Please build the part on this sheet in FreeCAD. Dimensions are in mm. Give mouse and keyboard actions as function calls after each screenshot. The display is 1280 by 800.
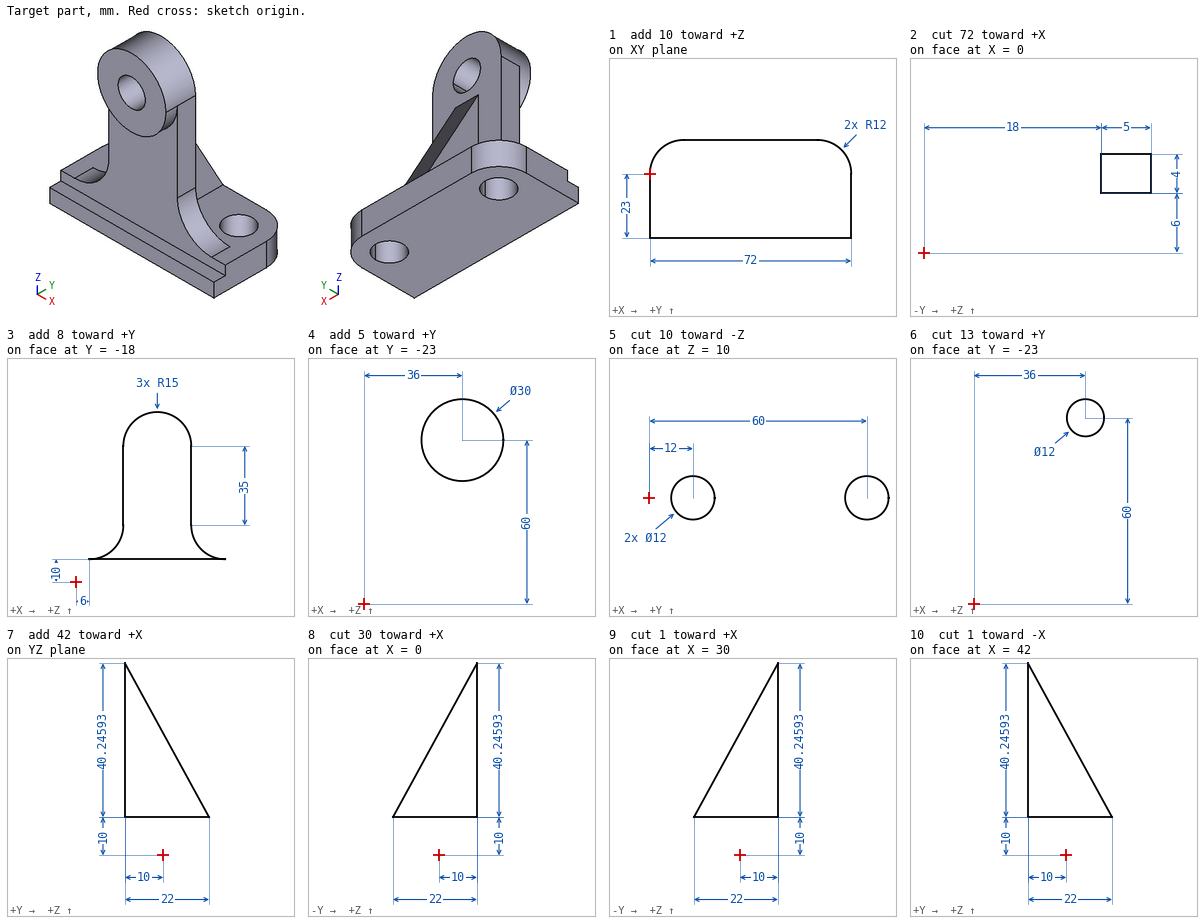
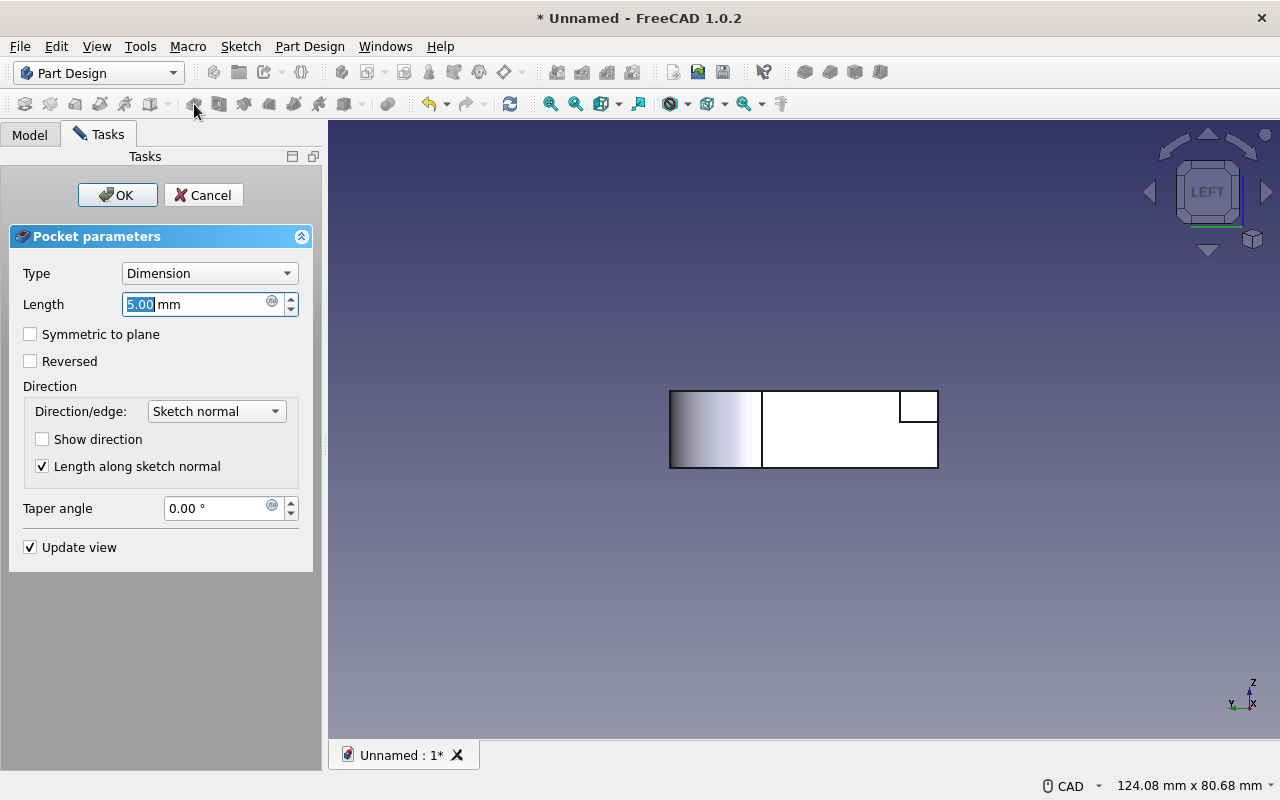
text(72)
key(Tab)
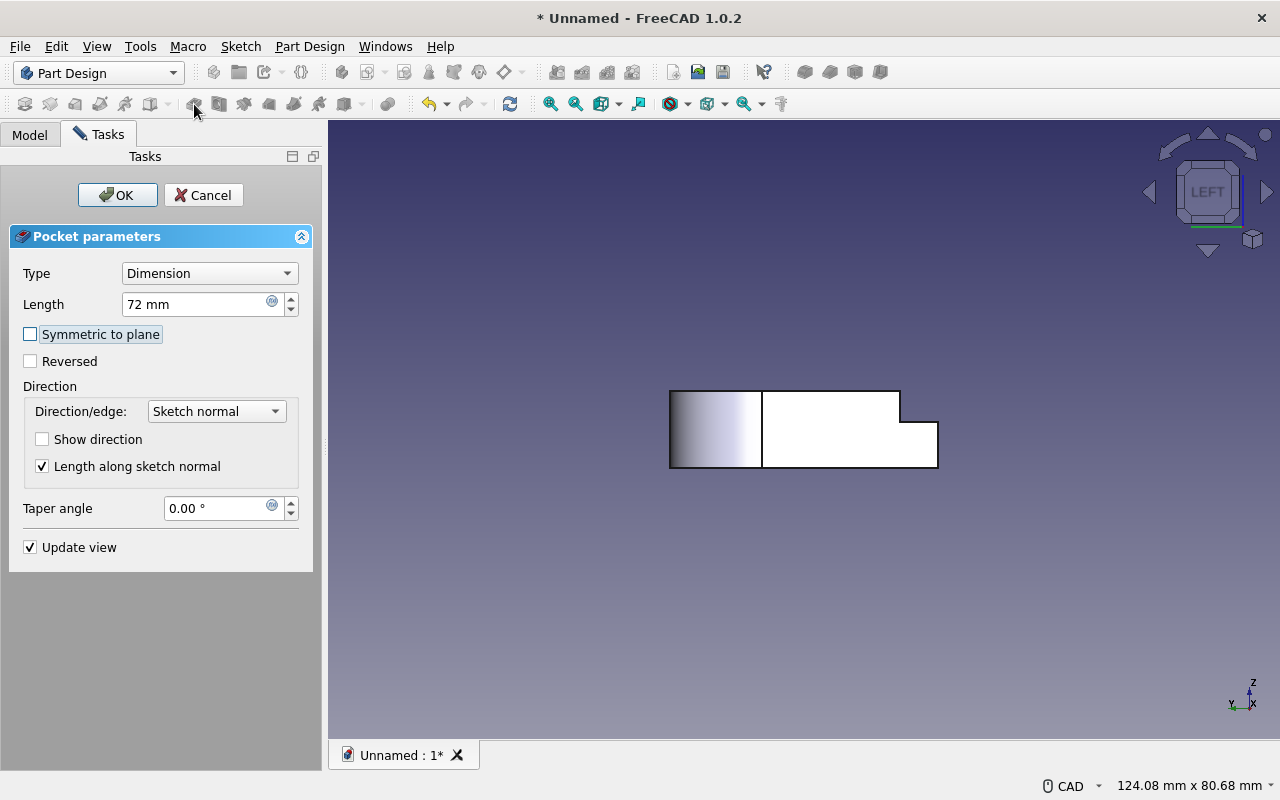
click(118, 195)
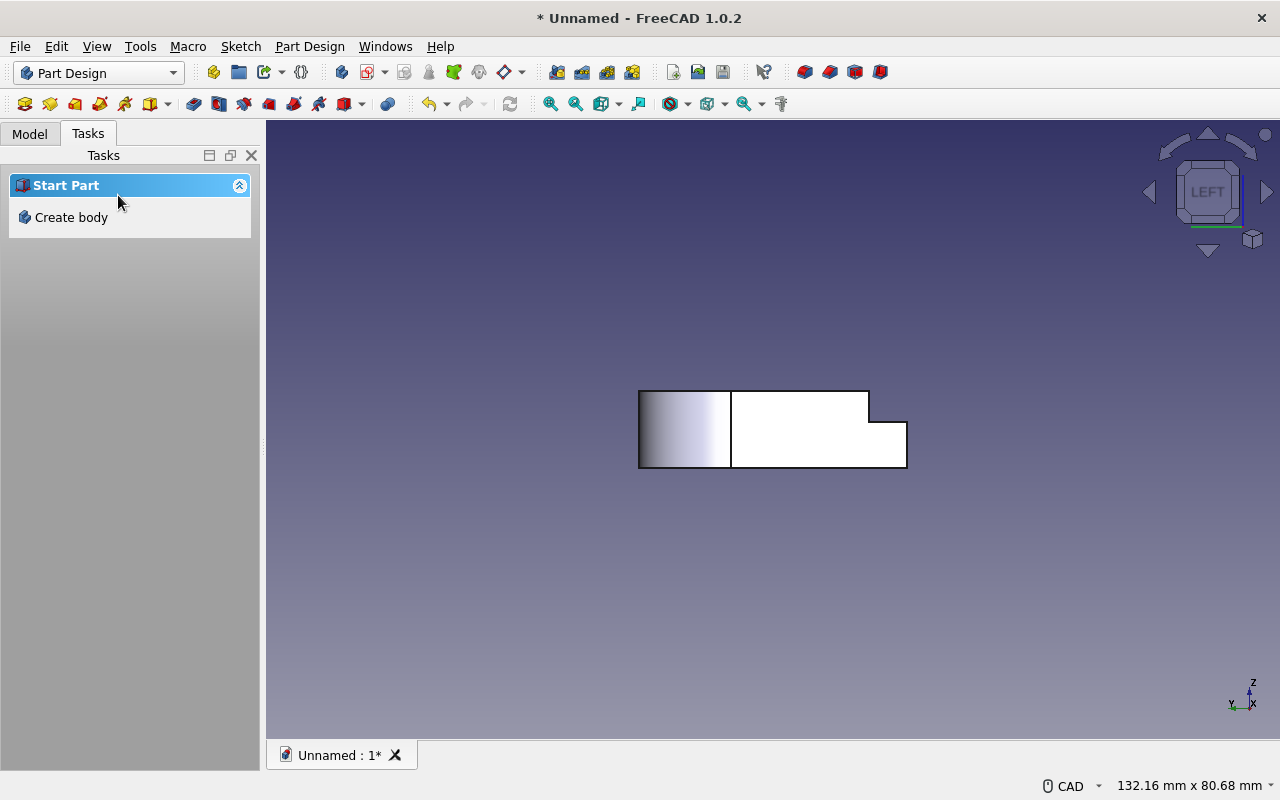
click(551, 104)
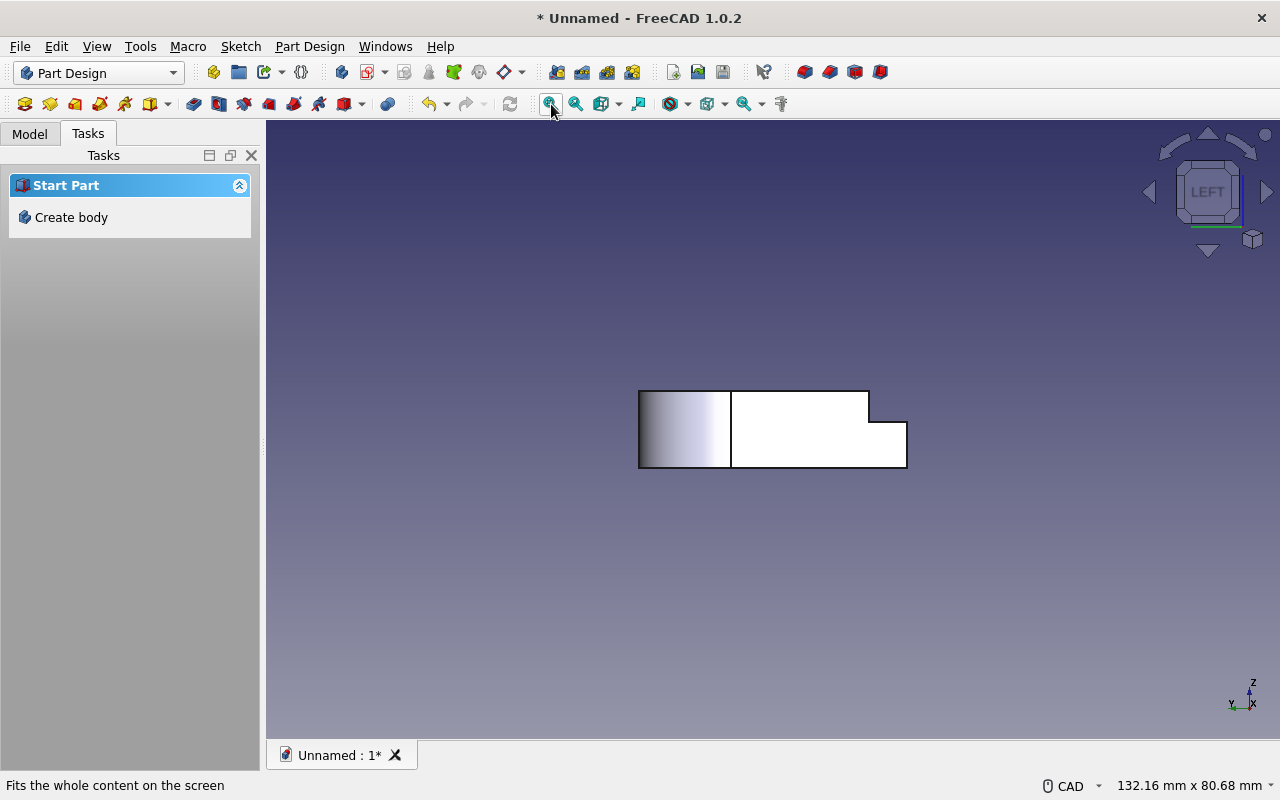
key(0)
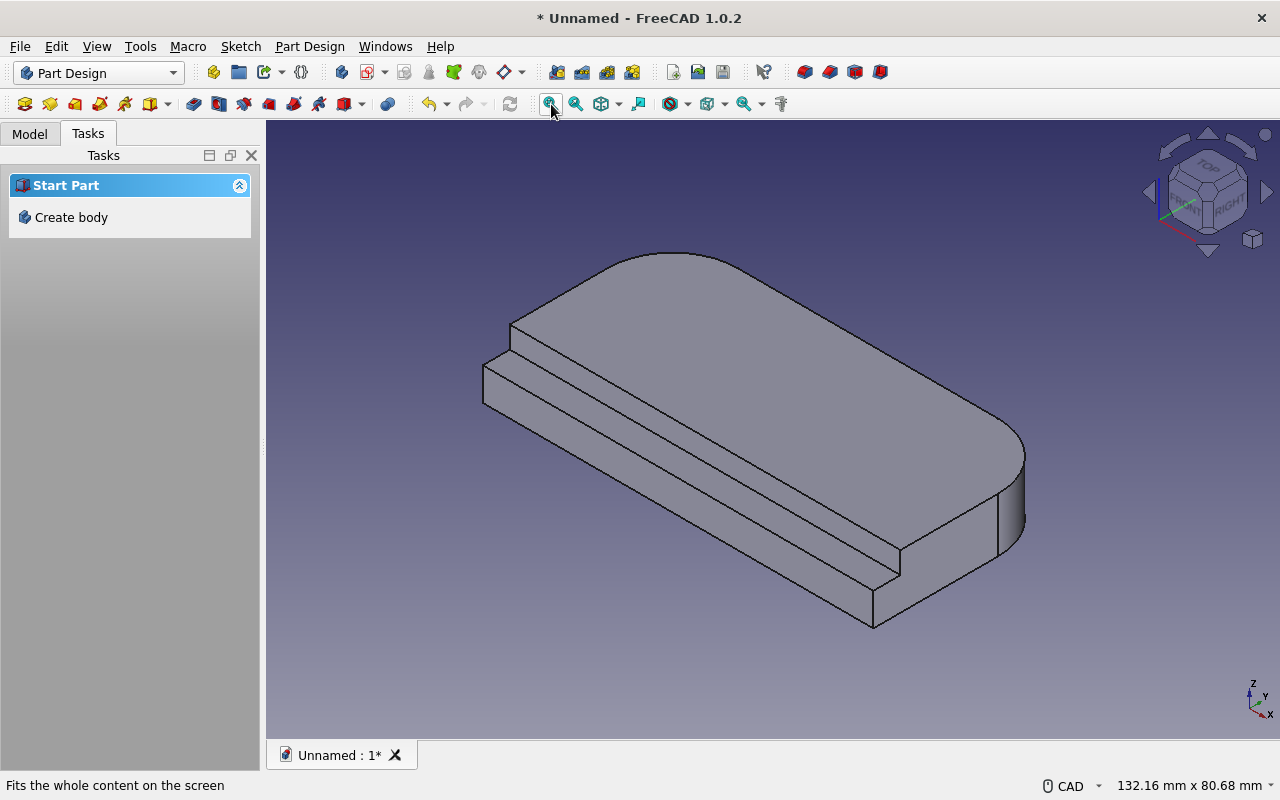
click(873, 546)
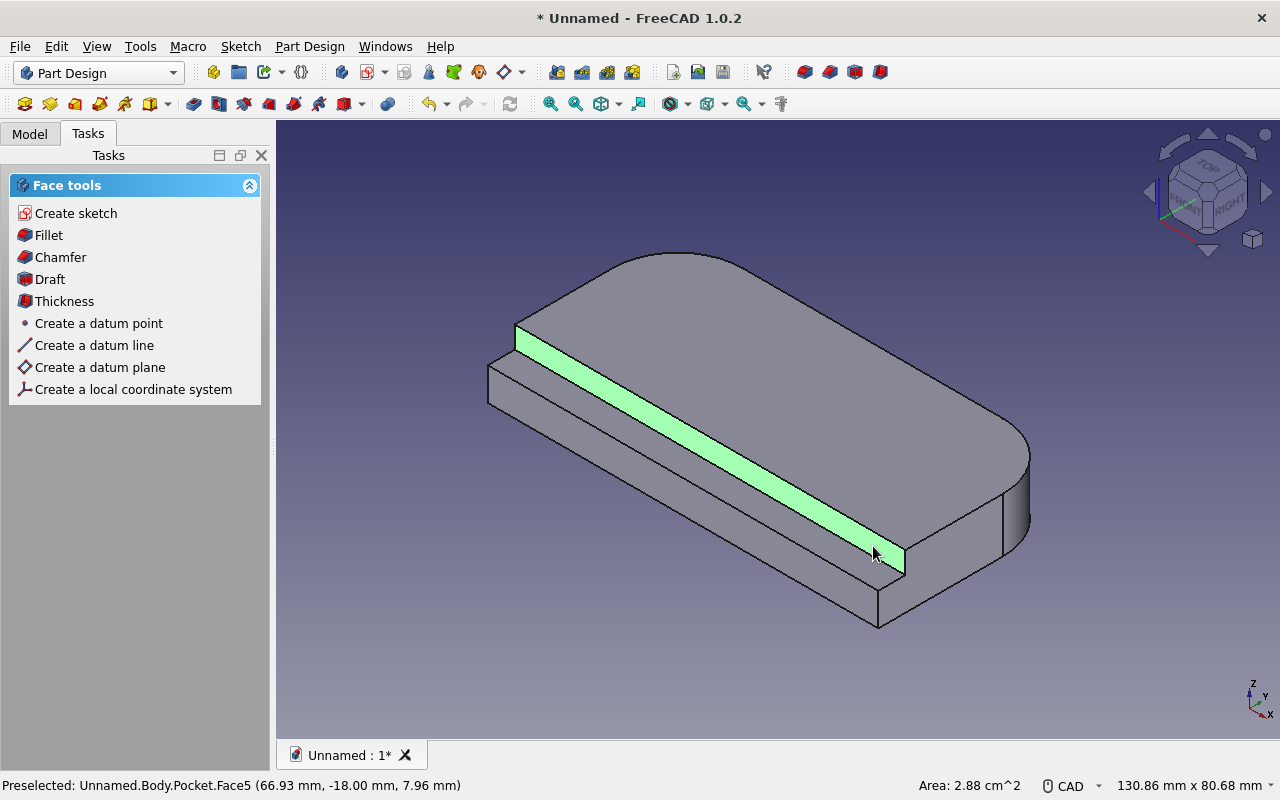
click(366, 72)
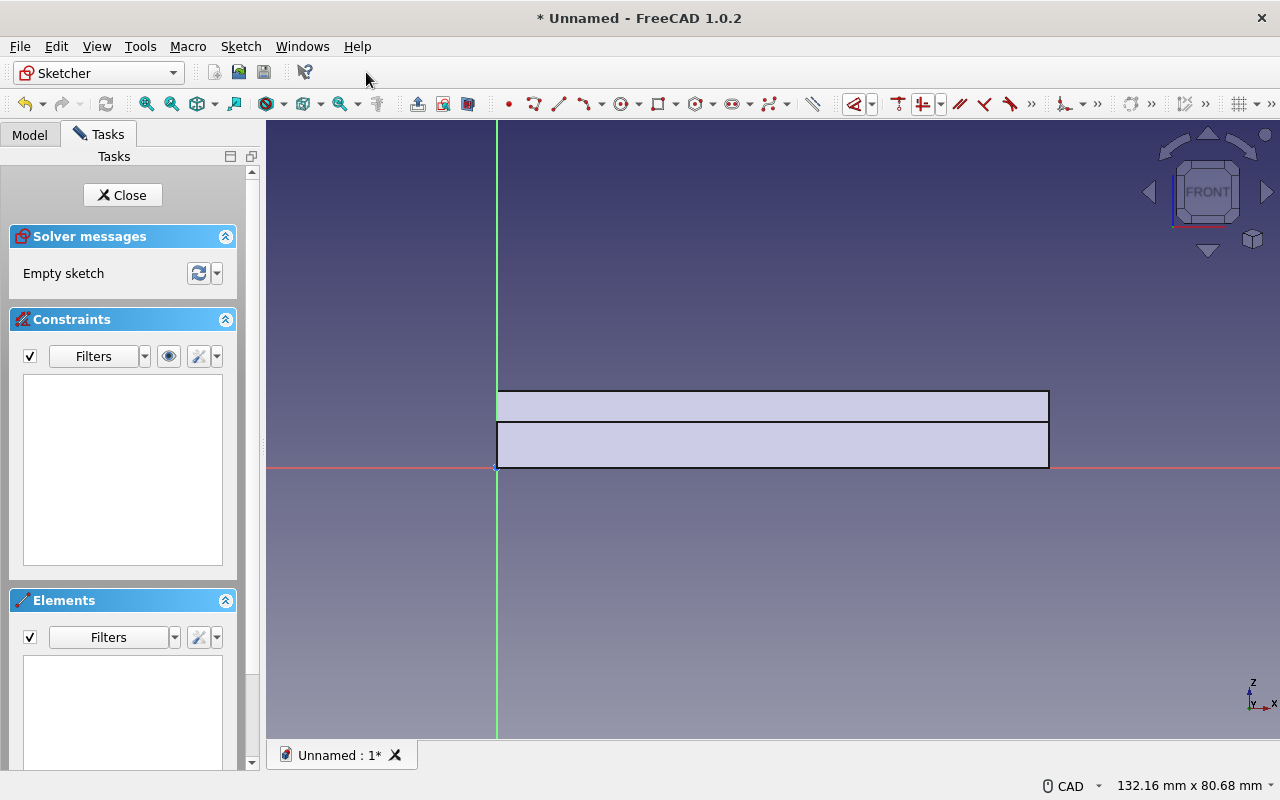
key(q)
key(s)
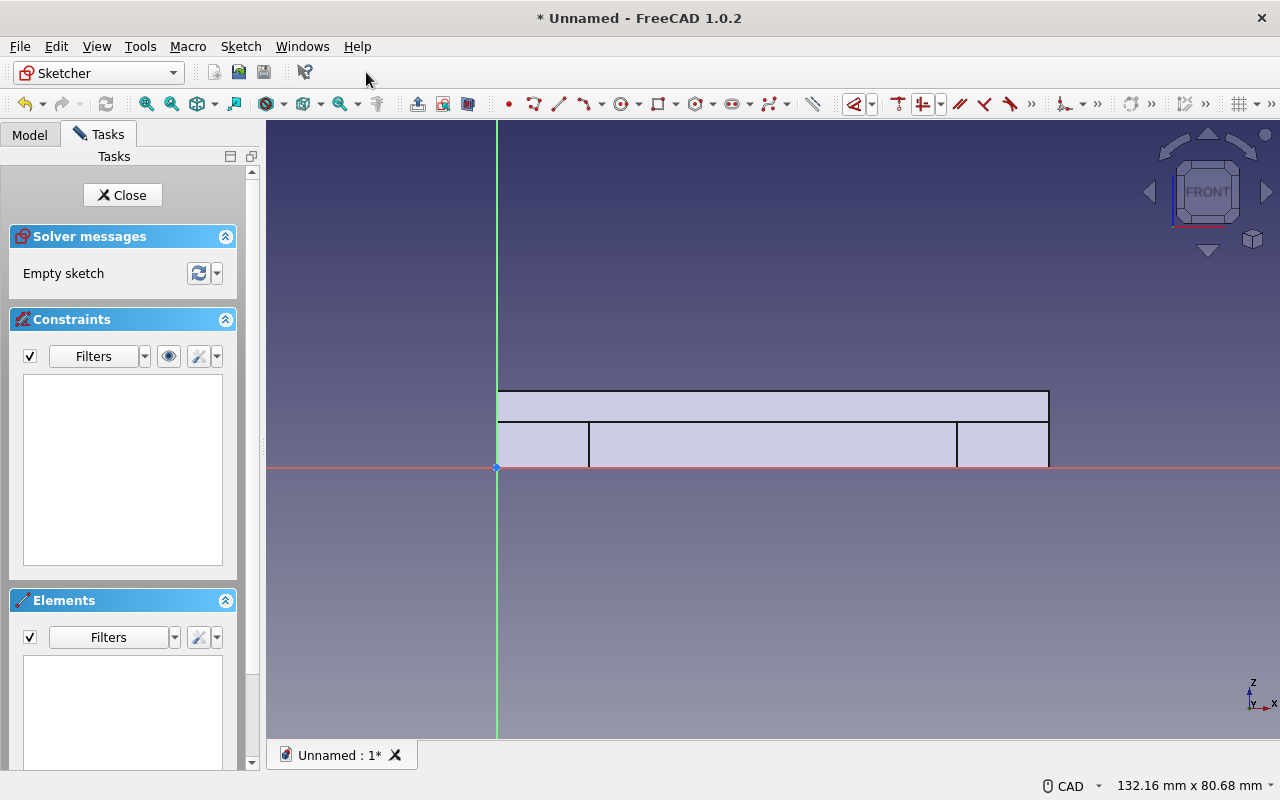
scroll(649, 711, down, 3)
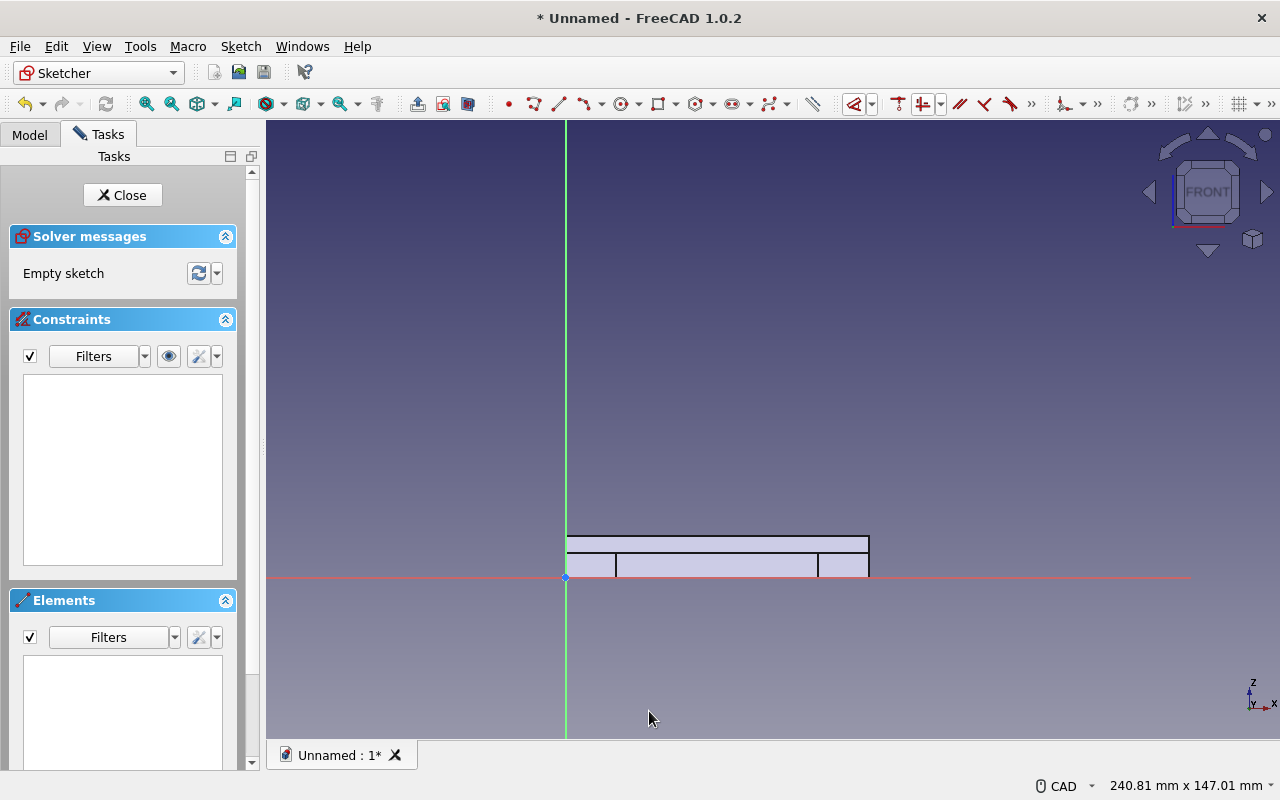
click(559, 104)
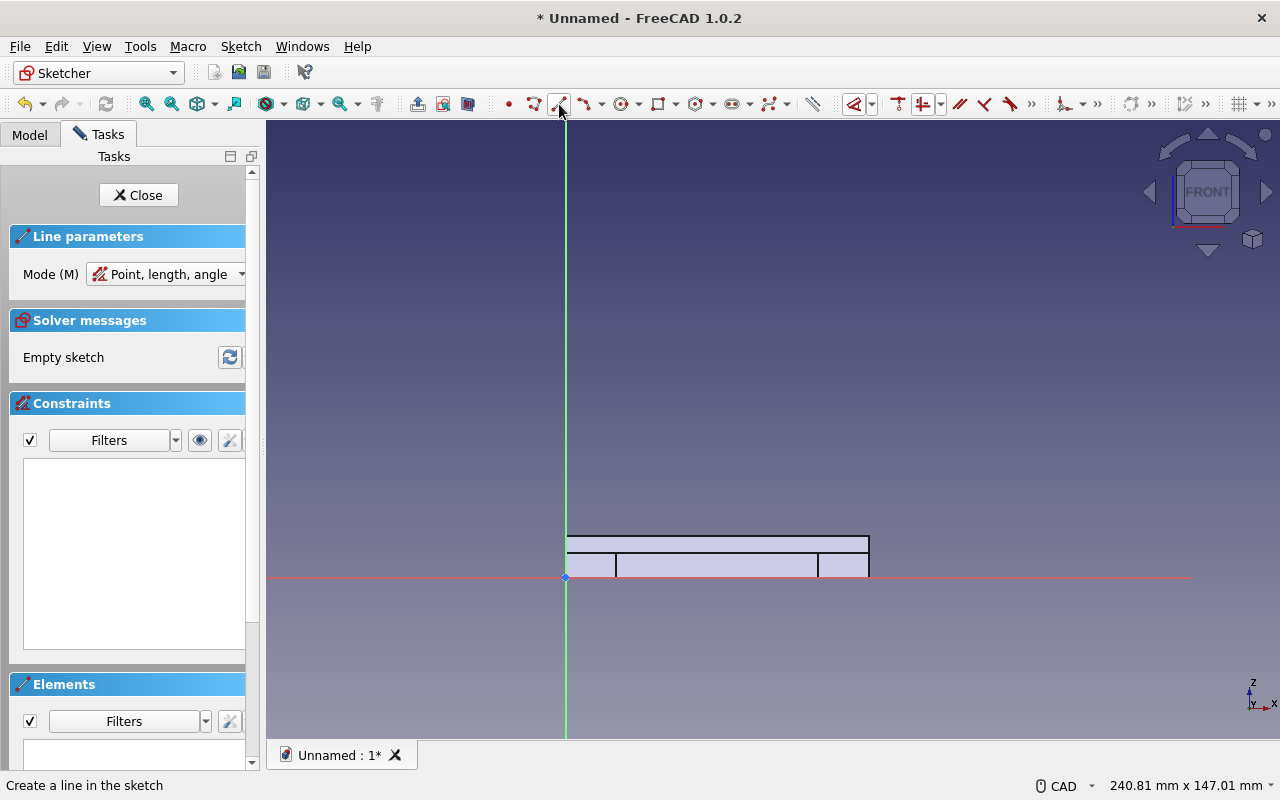
click(591, 536)
click(844, 536)